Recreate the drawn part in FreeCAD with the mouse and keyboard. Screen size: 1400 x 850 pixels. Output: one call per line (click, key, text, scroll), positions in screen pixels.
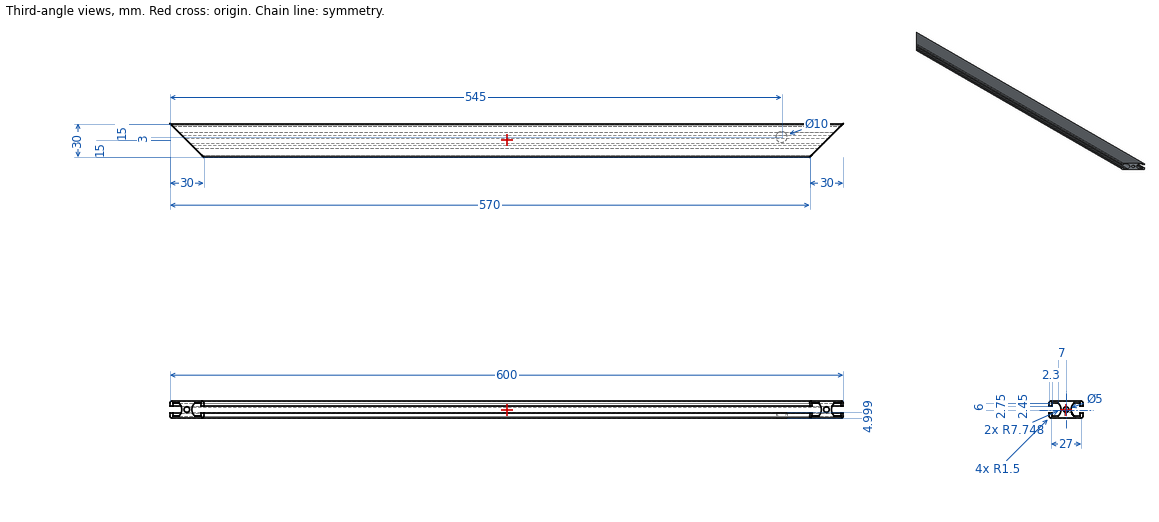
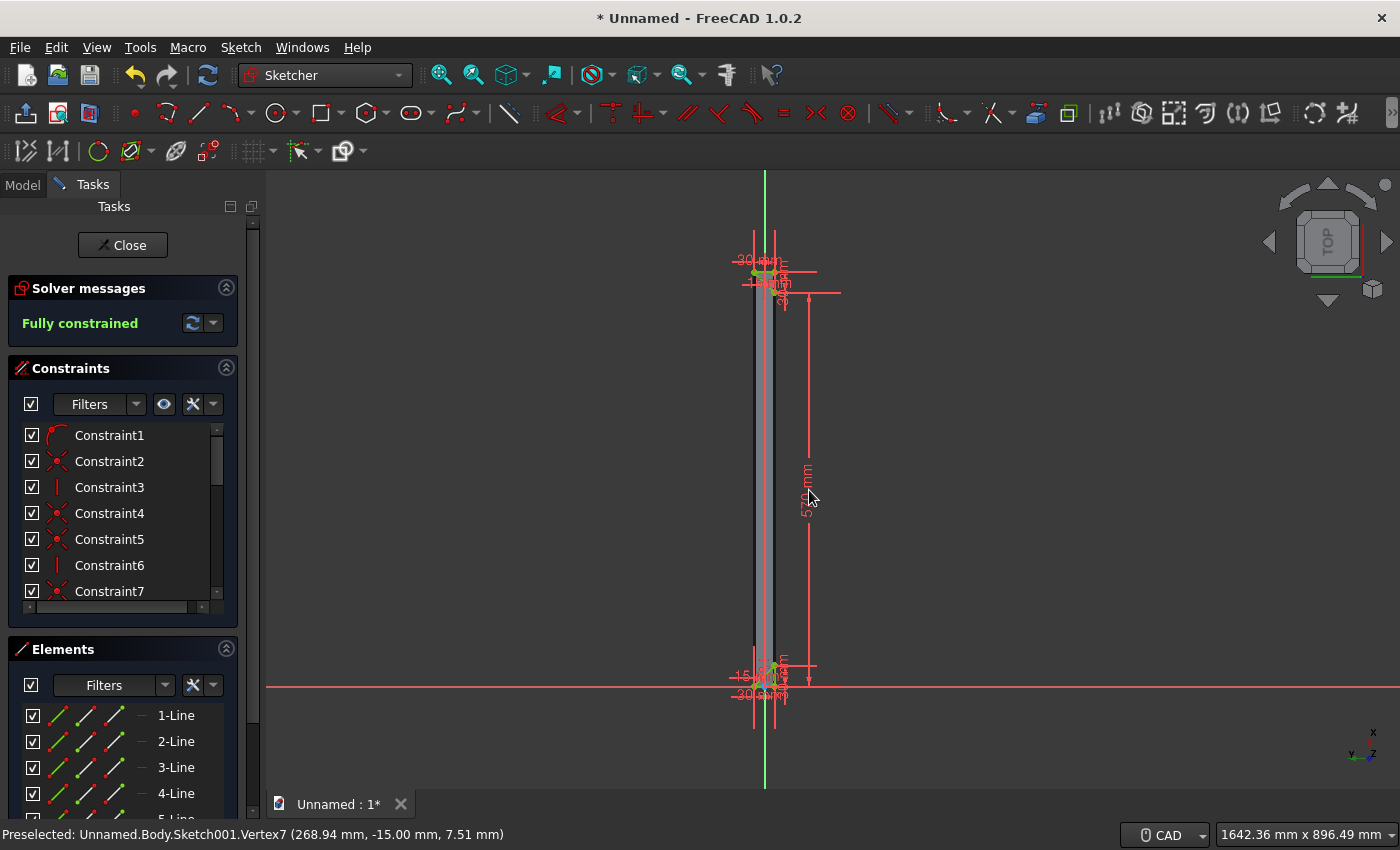
click(123, 245)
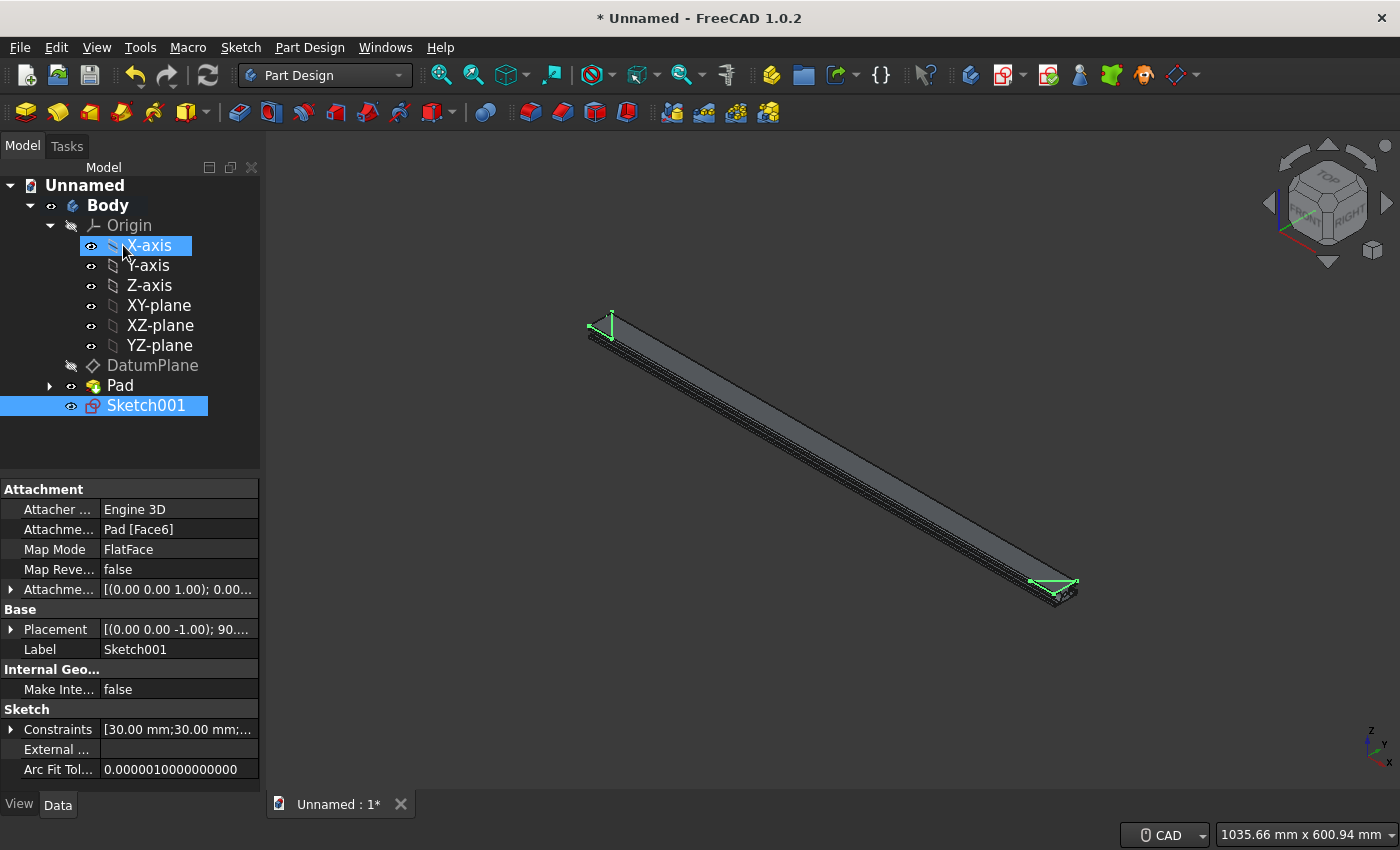
click(240, 112)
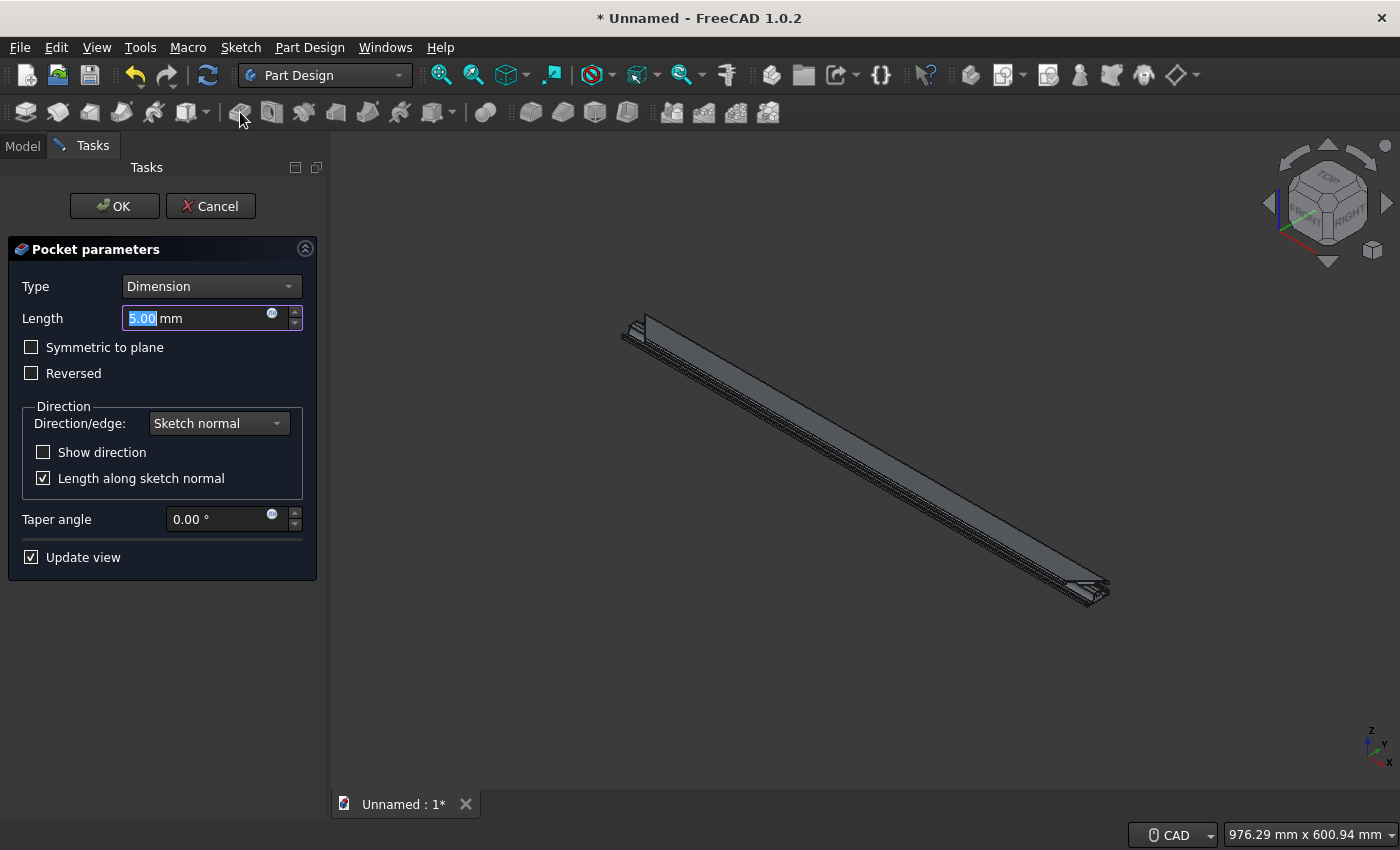
click(212, 286)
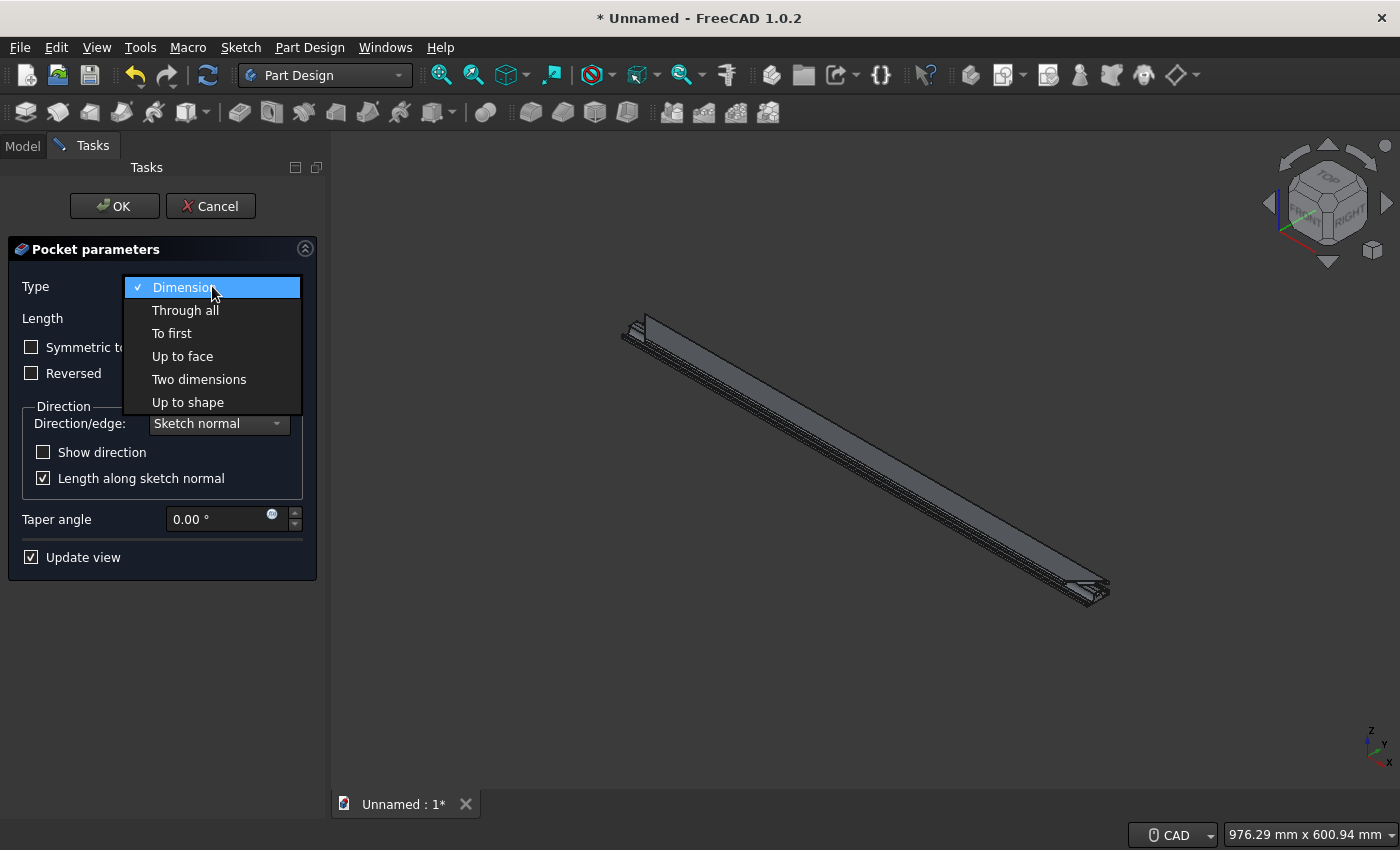
click(212, 310)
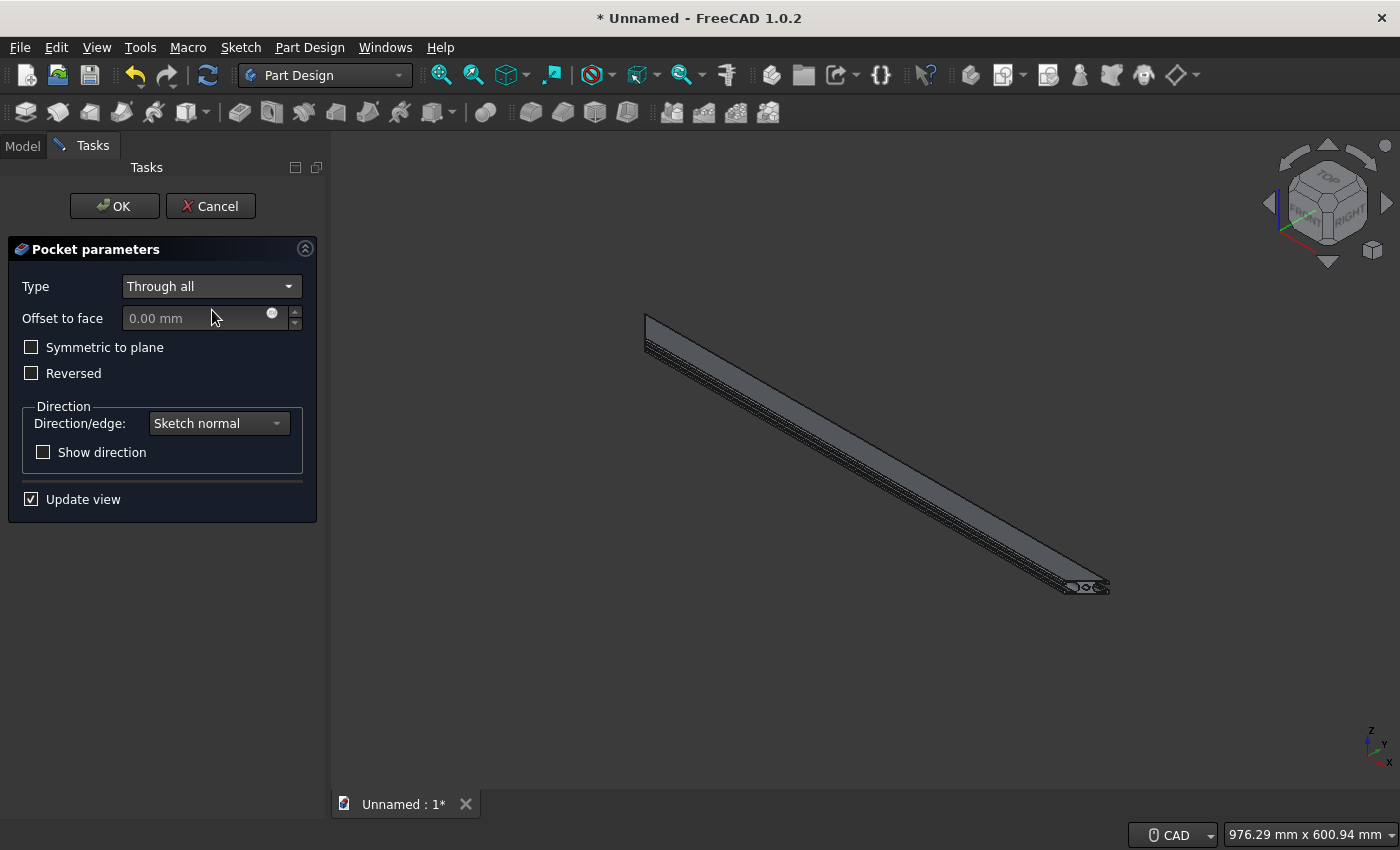
click(115, 206)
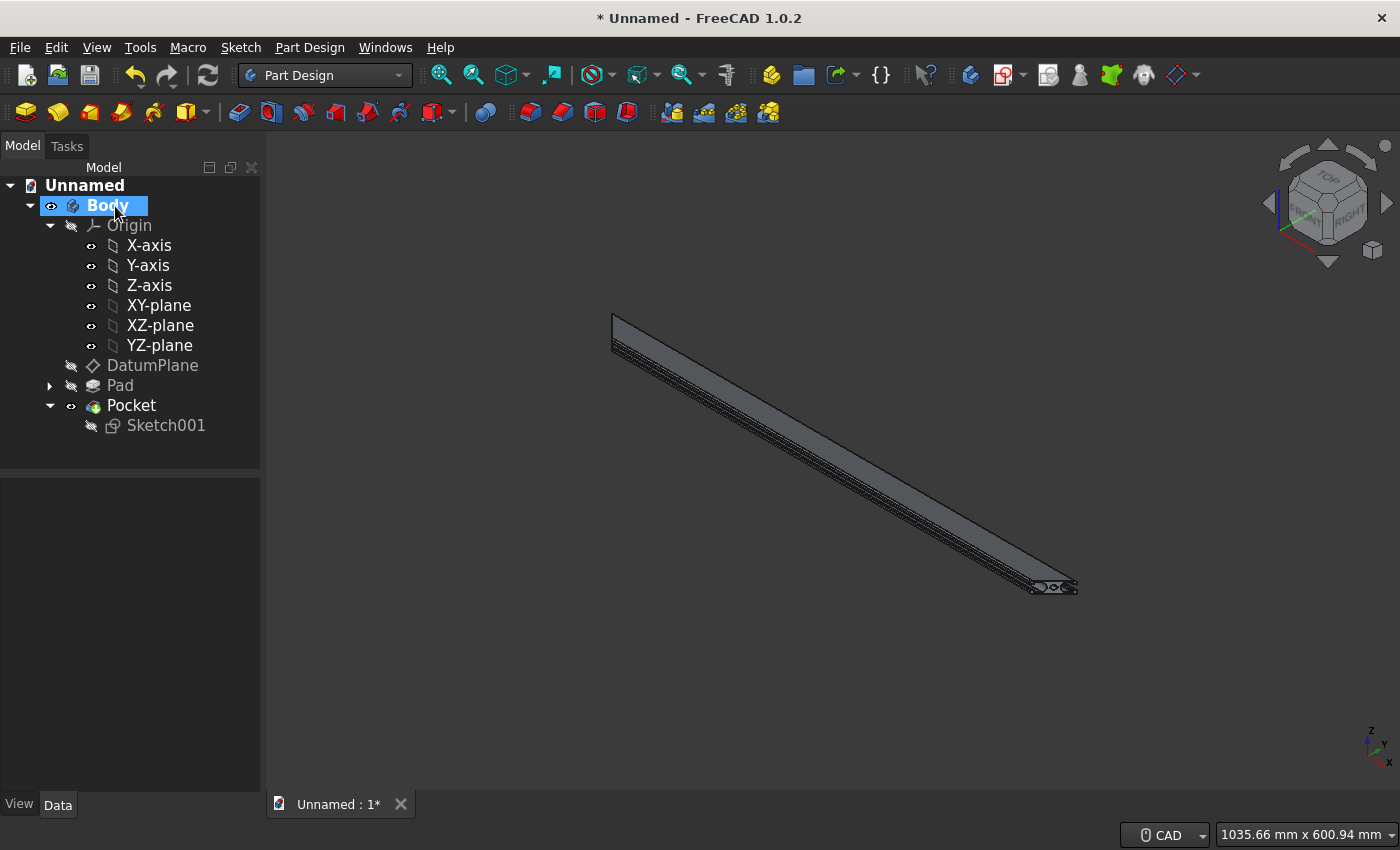
key(v)
key(f)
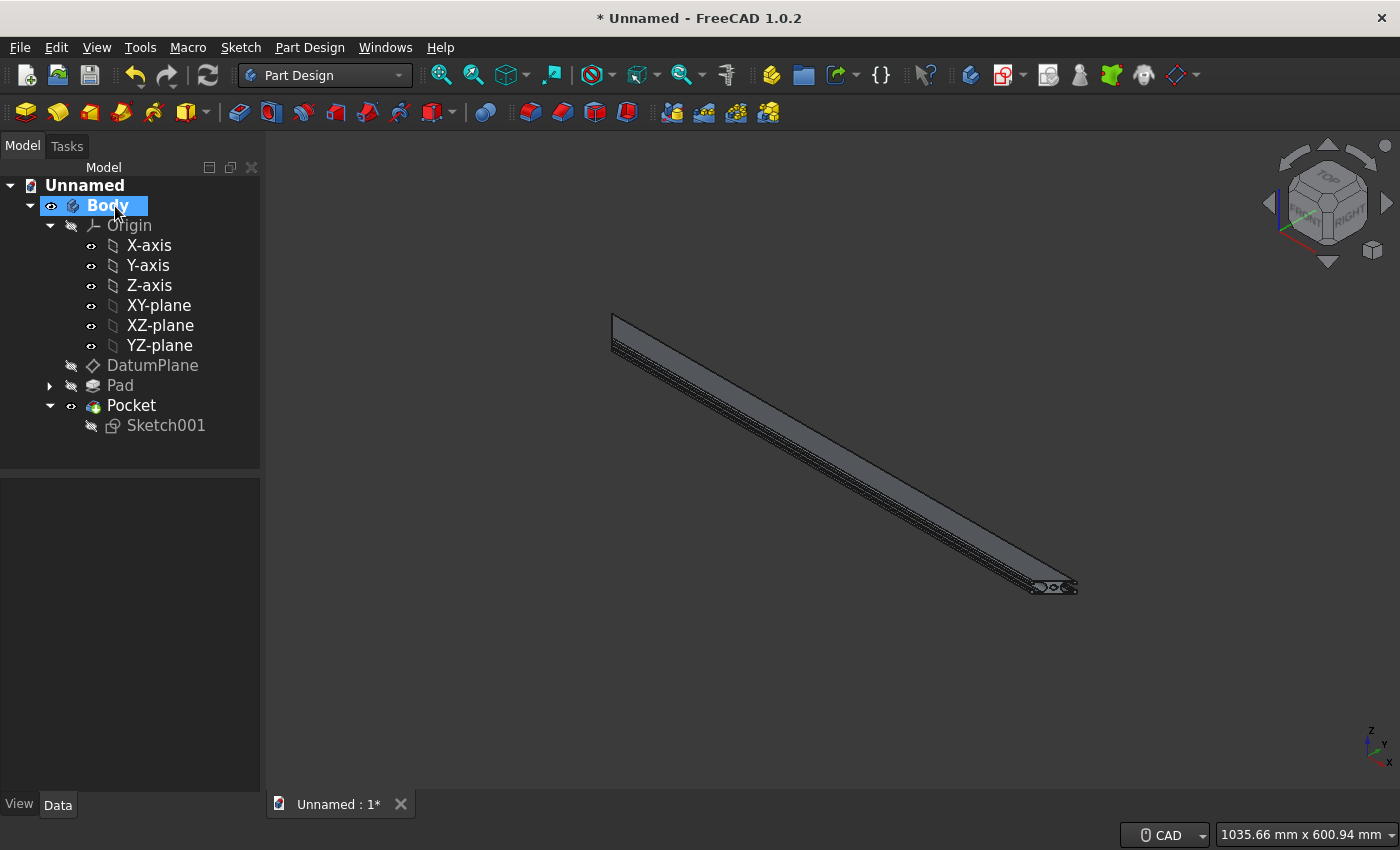
key(5)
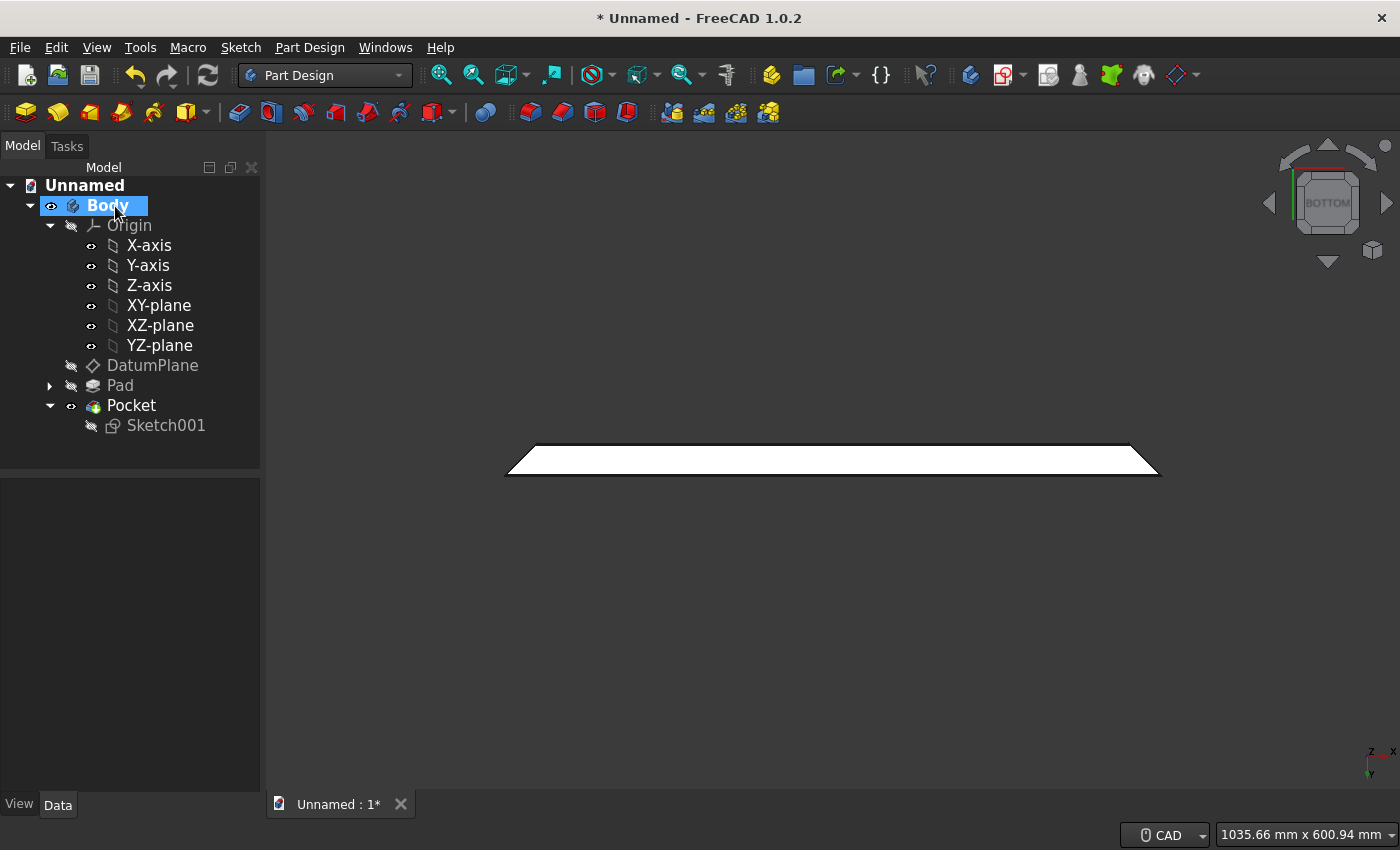
click(833, 459)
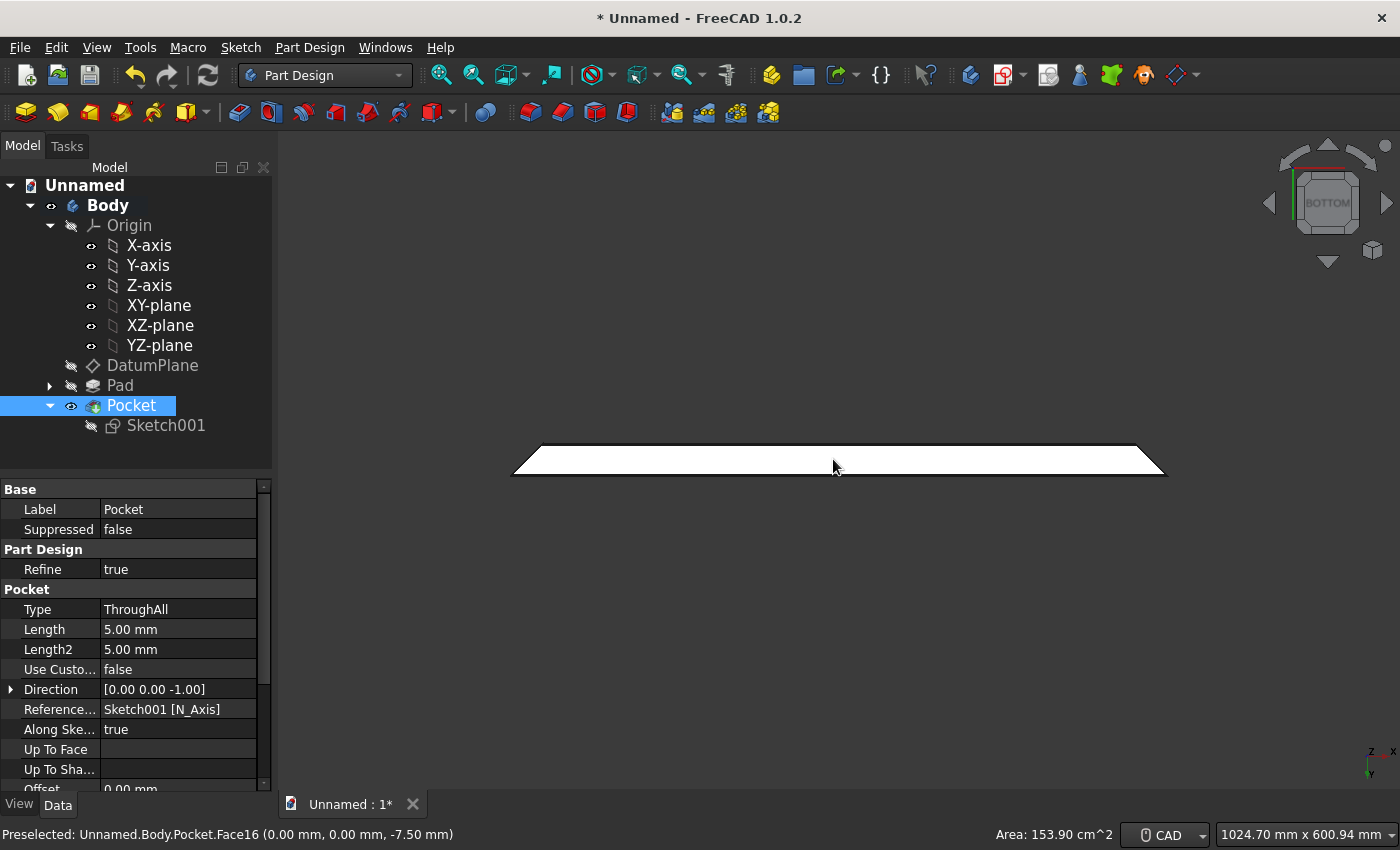
click(1004, 76)